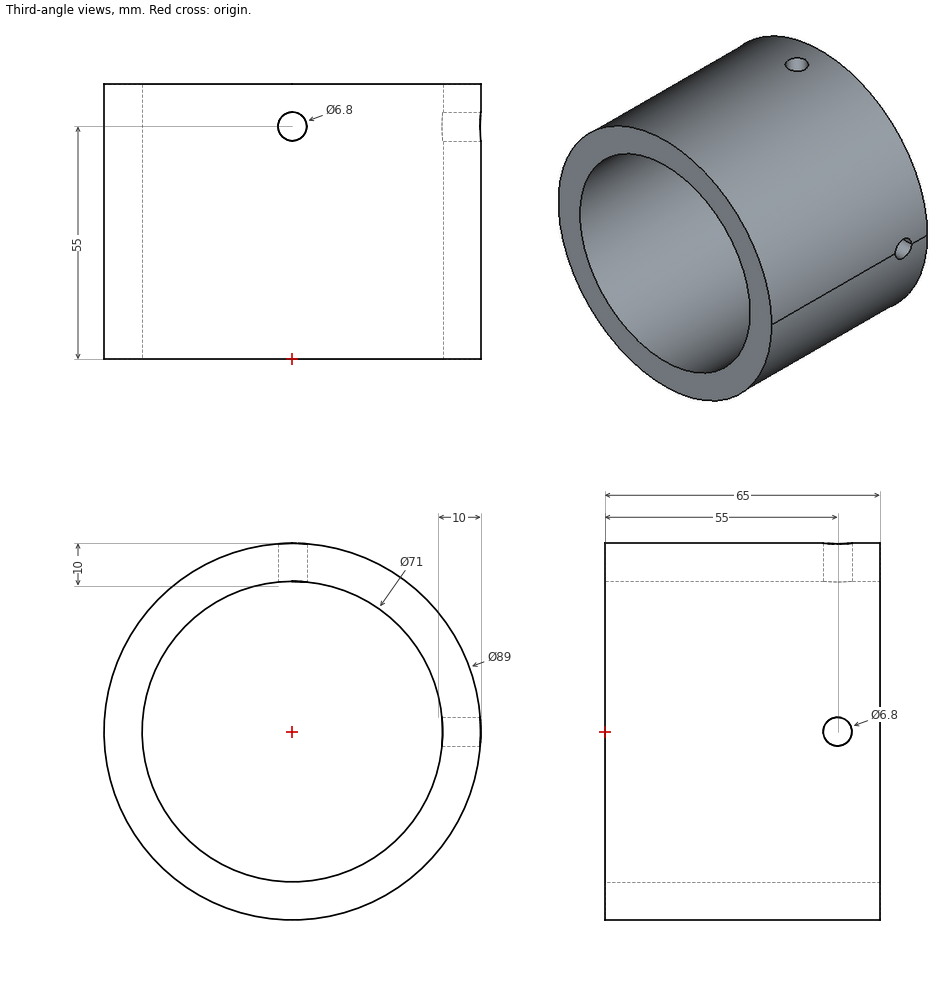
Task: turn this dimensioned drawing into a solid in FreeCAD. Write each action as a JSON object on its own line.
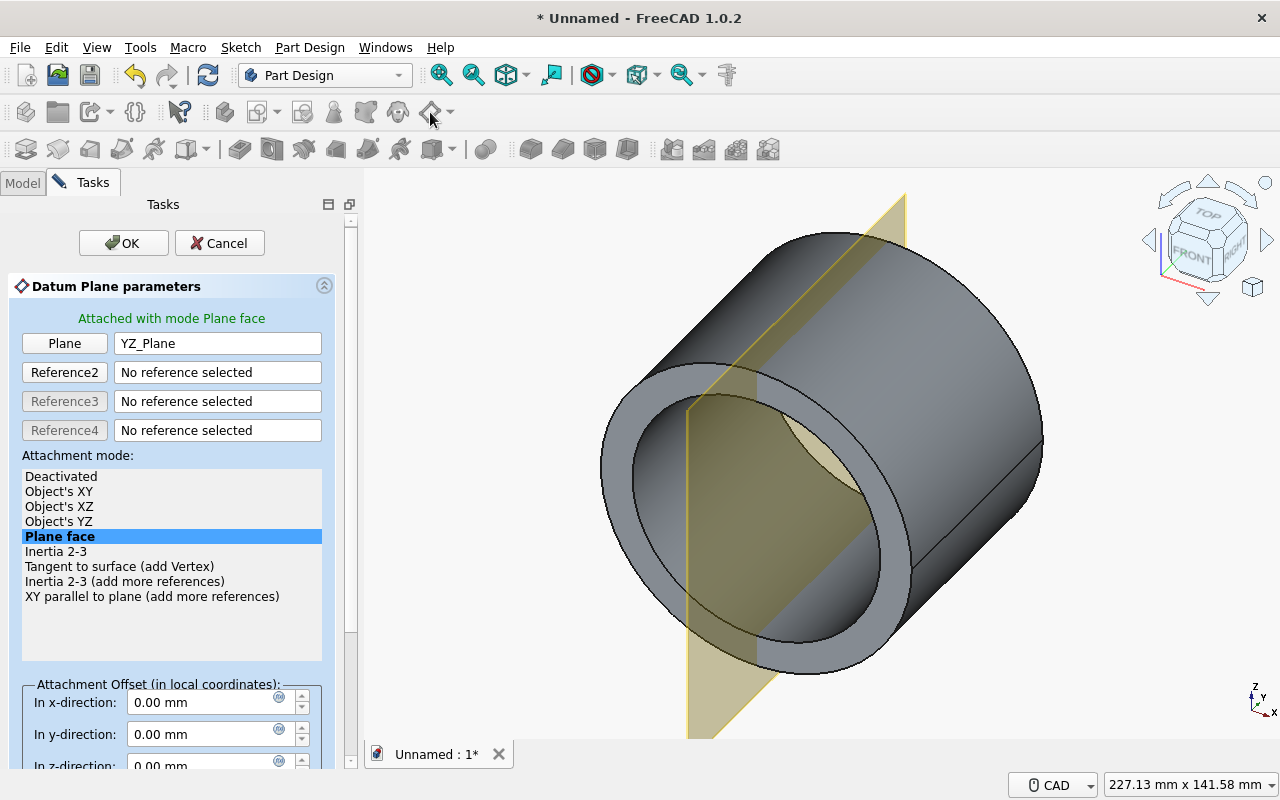
{"action": "scroll", "coordinate": [351, 491], "scroll_direction": "down", "scroll_amount": 2}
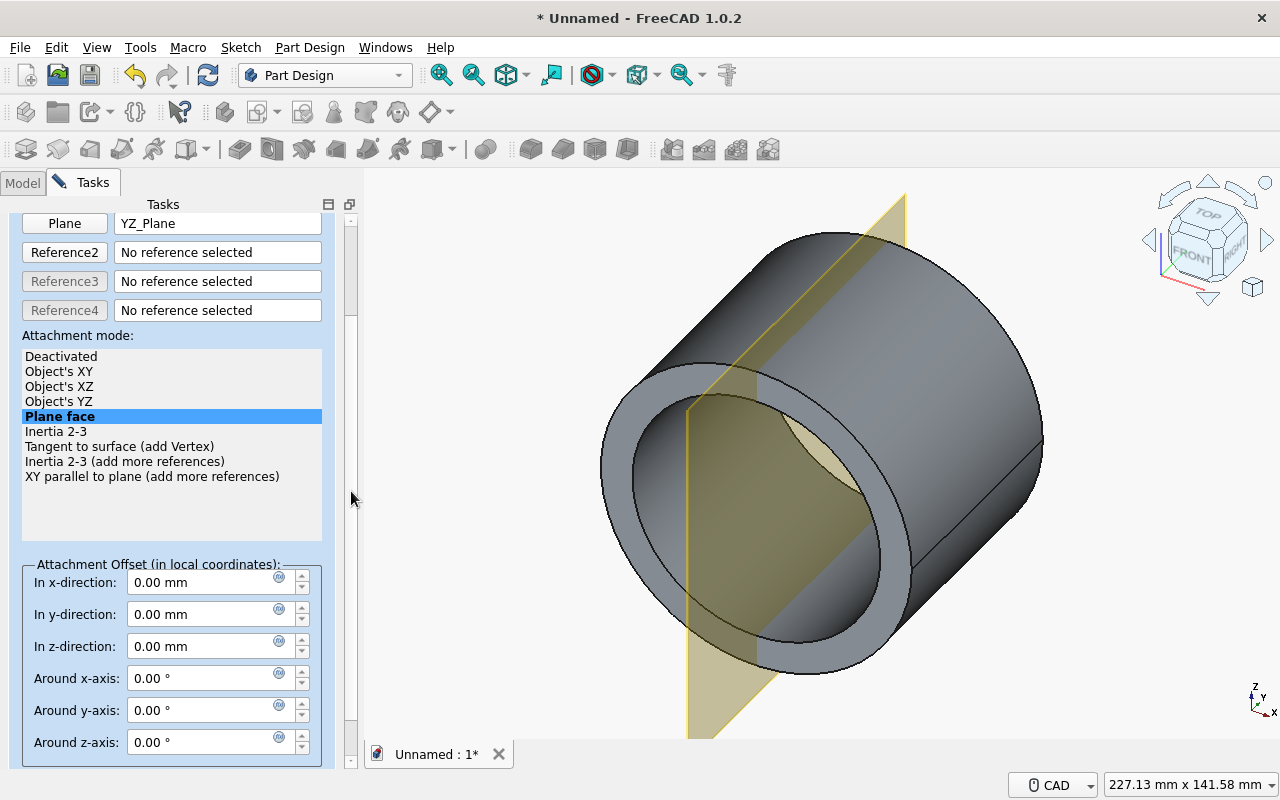
{"action": "triple_click", "coordinate": [210, 646]}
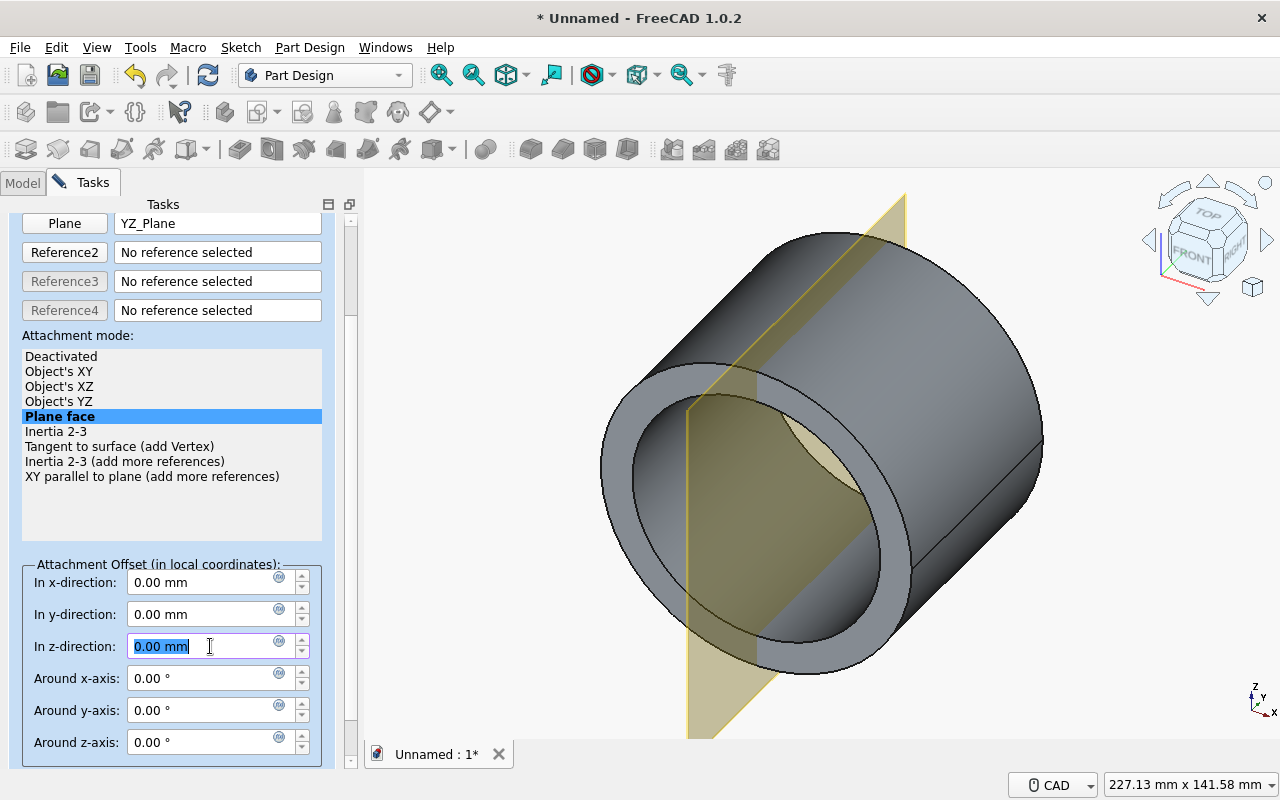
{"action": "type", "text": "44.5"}
{"action": "key", "text": "Tab"}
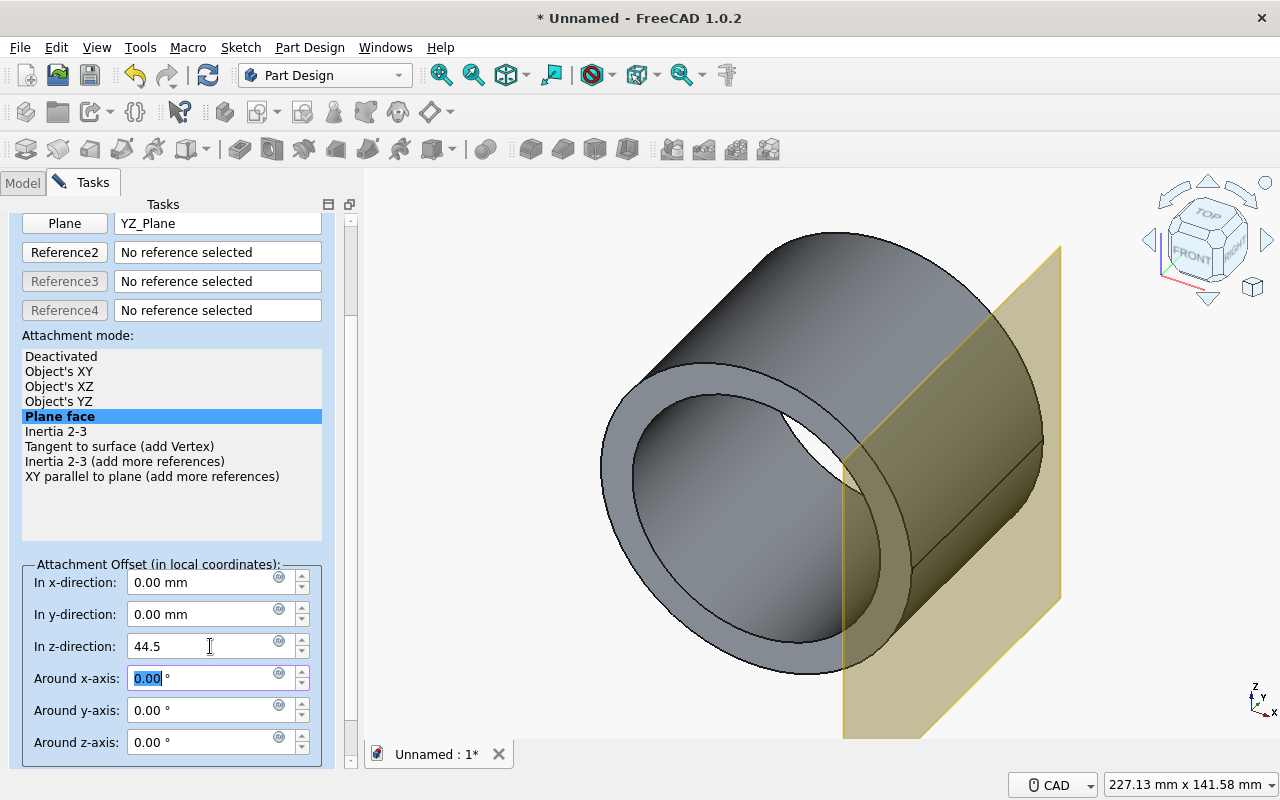
{"action": "scroll", "coordinate": [351, 491], "scroll_direction": "up", "scroll_amount": 3}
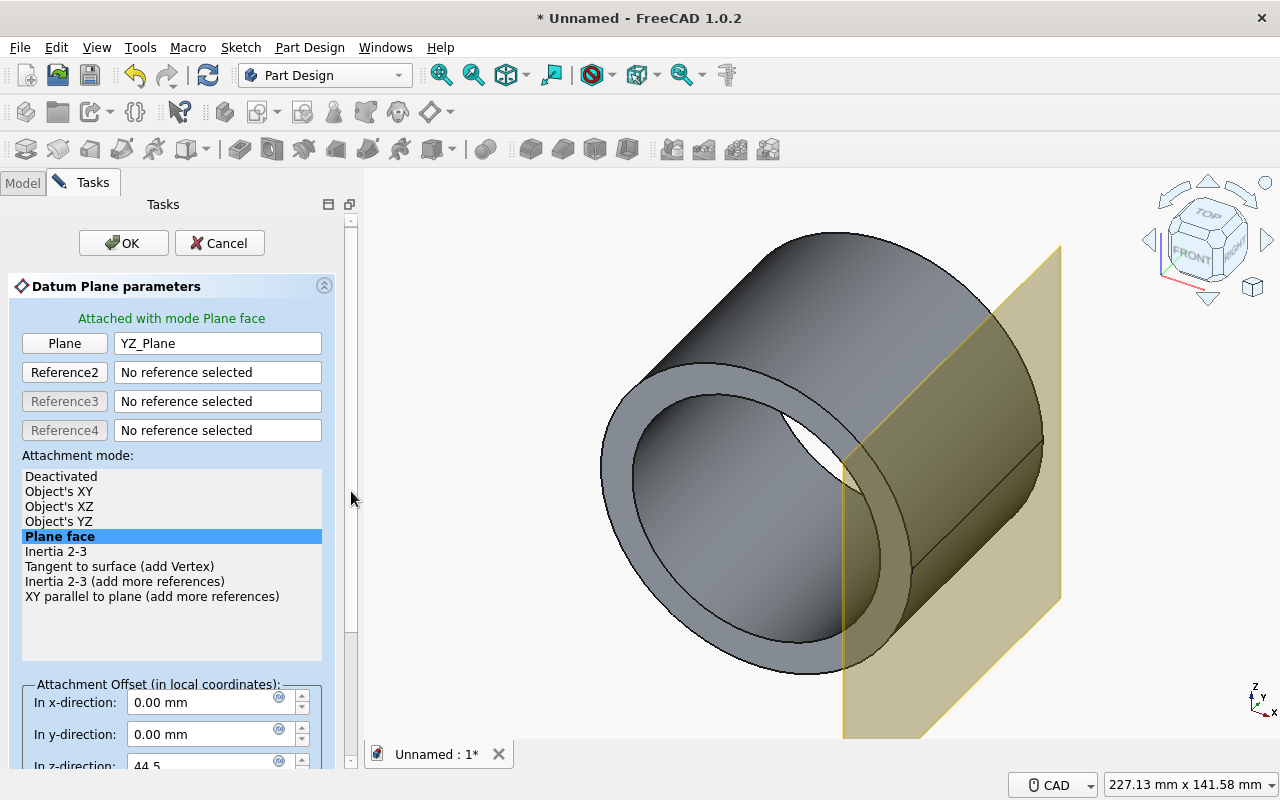
{"action": "left_click", "coordinate": [124, 243]}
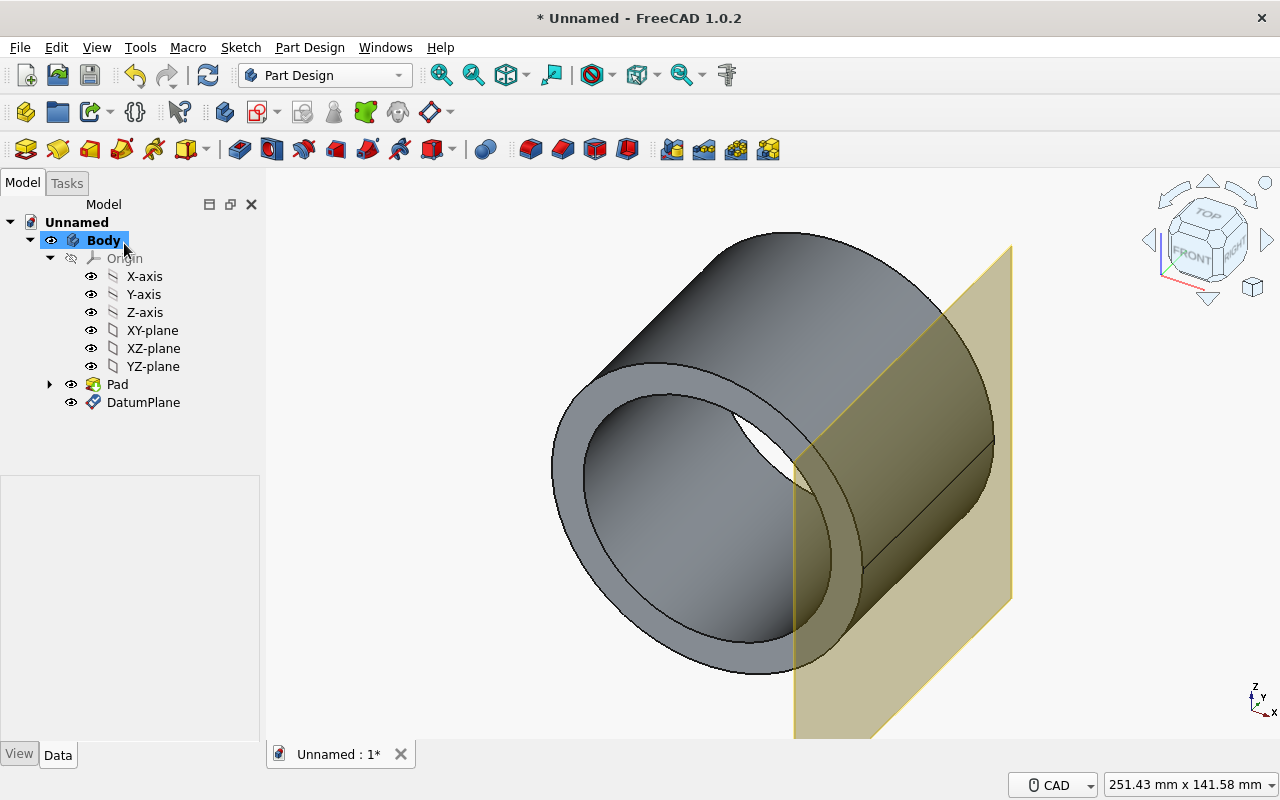
{"action": "left_click", "coordinate": [116, 402]}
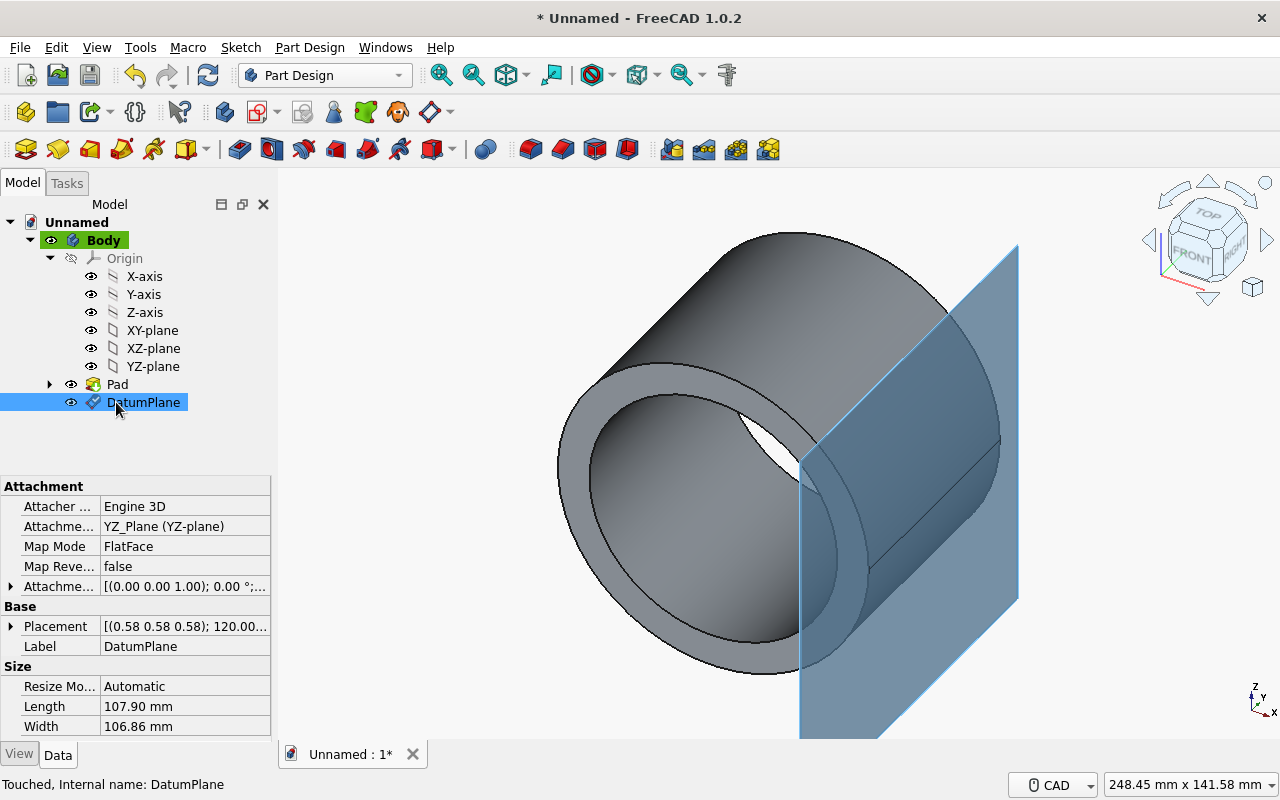
{"action": "left_click", "coordinate": [258, 112]}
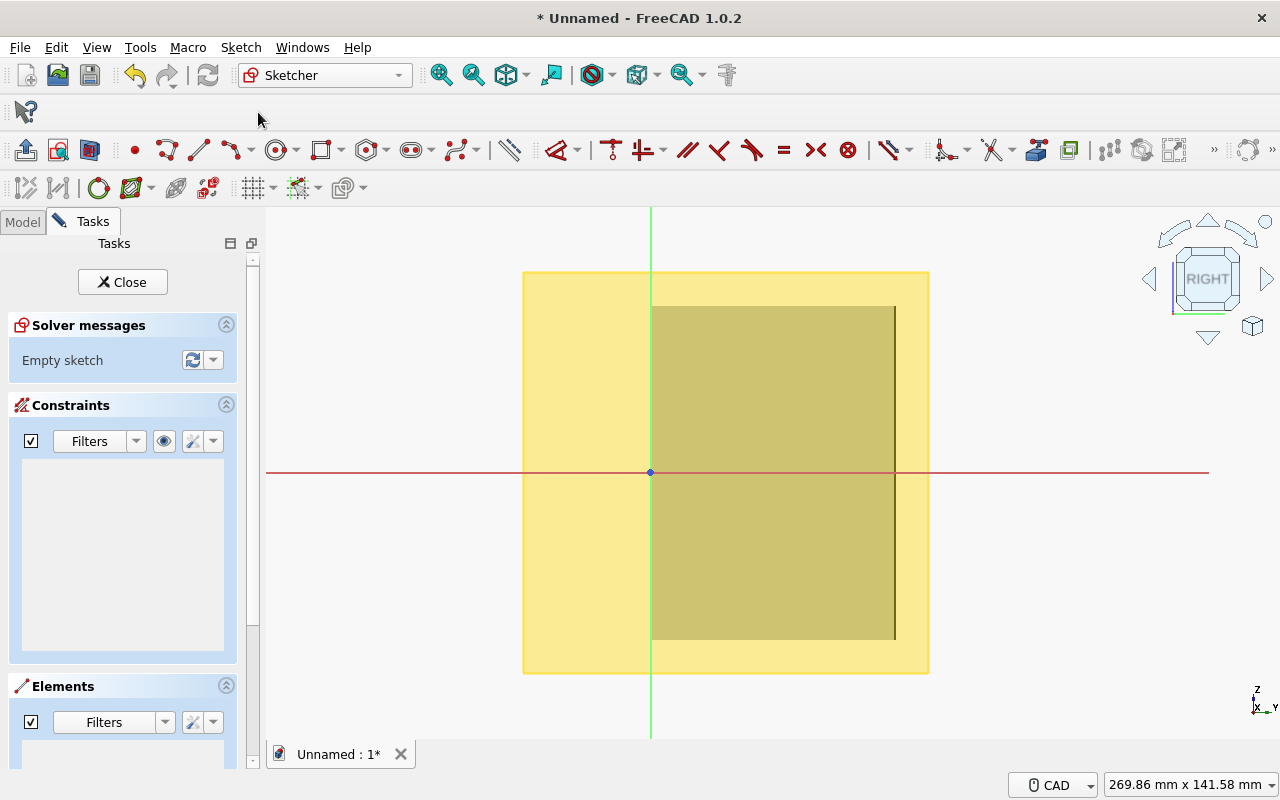
{"action": "scroll", "coordinate": [870, 473], "scroll_direction": "up", "scroll_amount": 13}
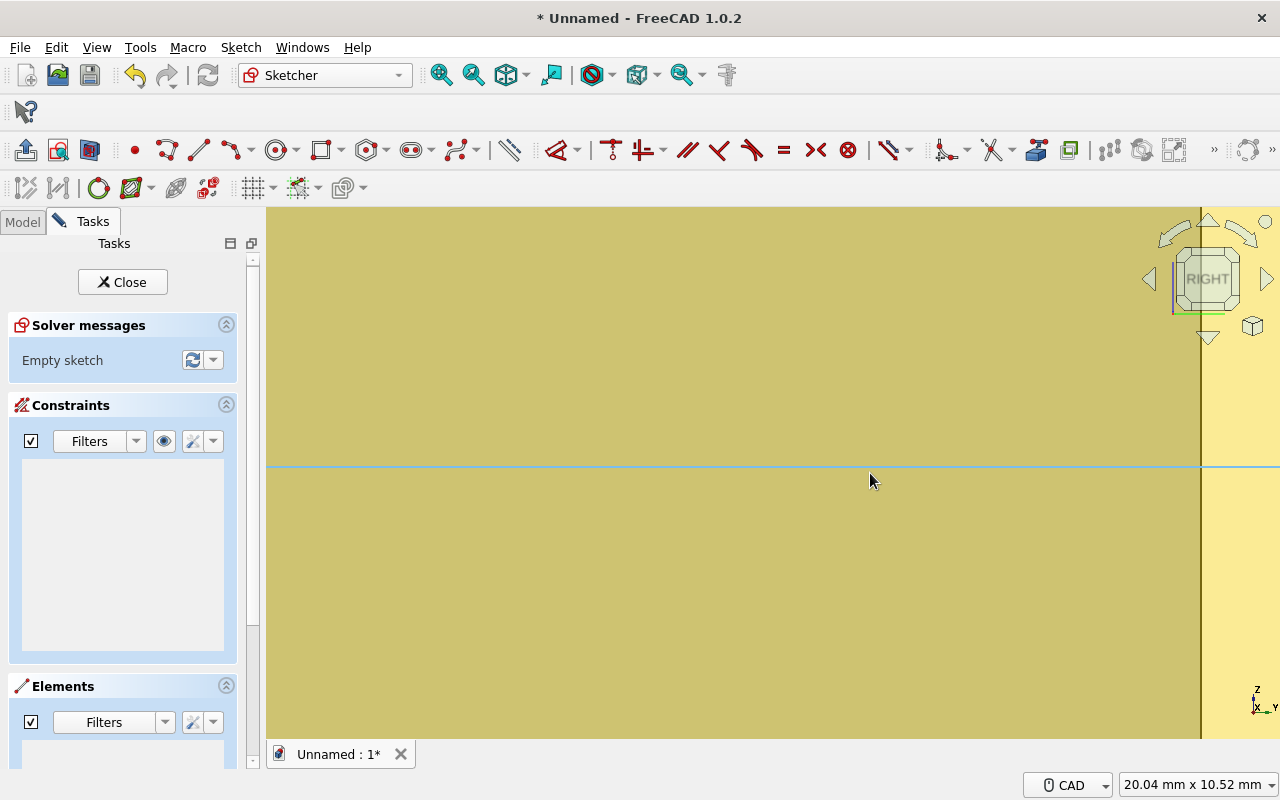
{"action": "key", "text": "g c"}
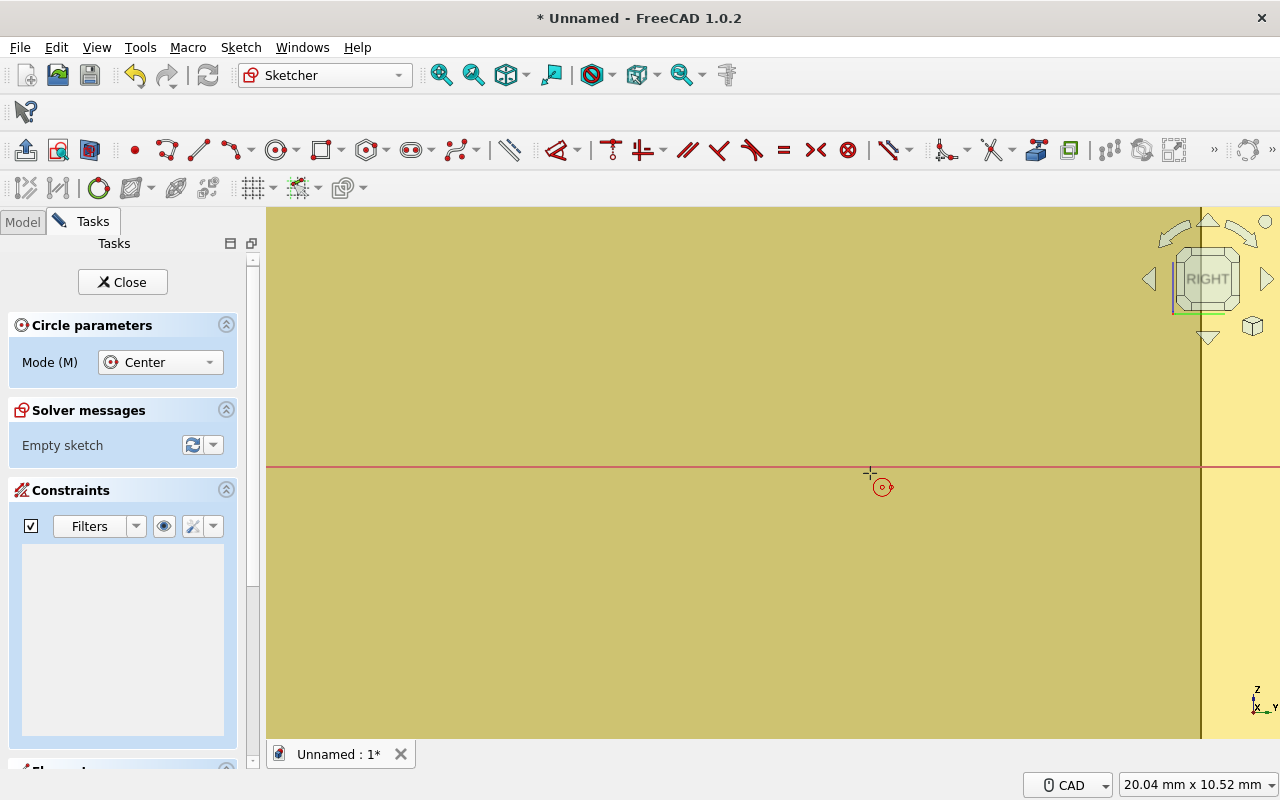
{"action": "left_click", "coordinate": [695, 467]}
{"action": "mouse_move", "coordinate": [816, 345]}